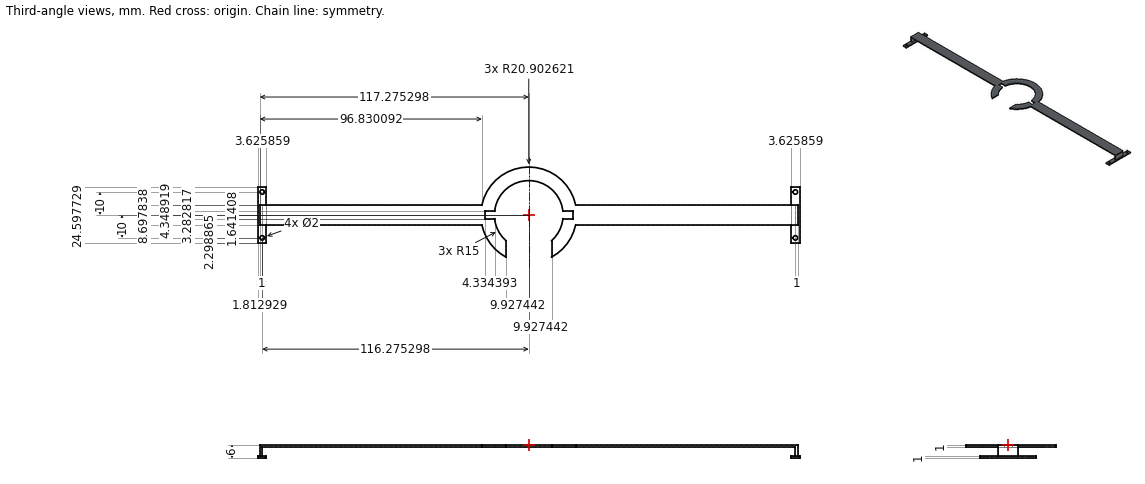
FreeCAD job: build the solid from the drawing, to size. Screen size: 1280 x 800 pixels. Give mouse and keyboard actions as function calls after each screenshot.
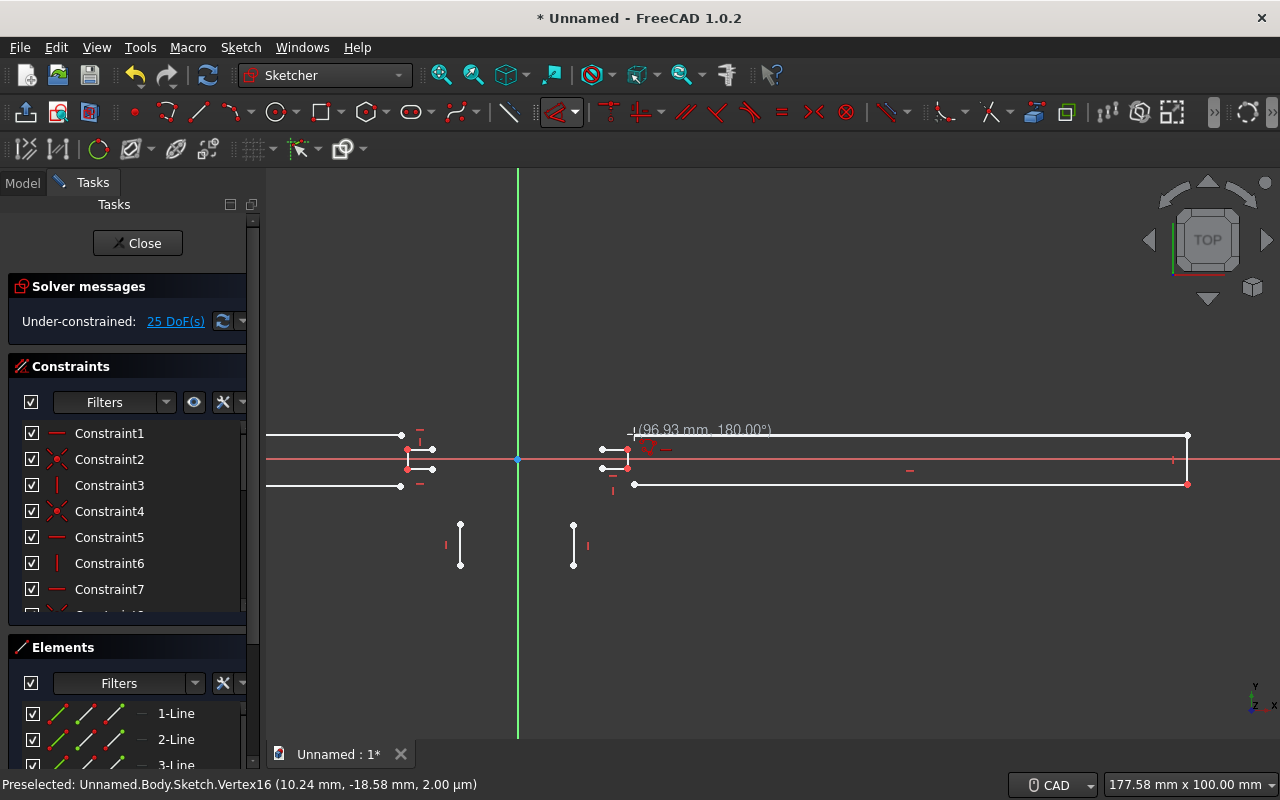
click(634, 434)
right_click(634, 434)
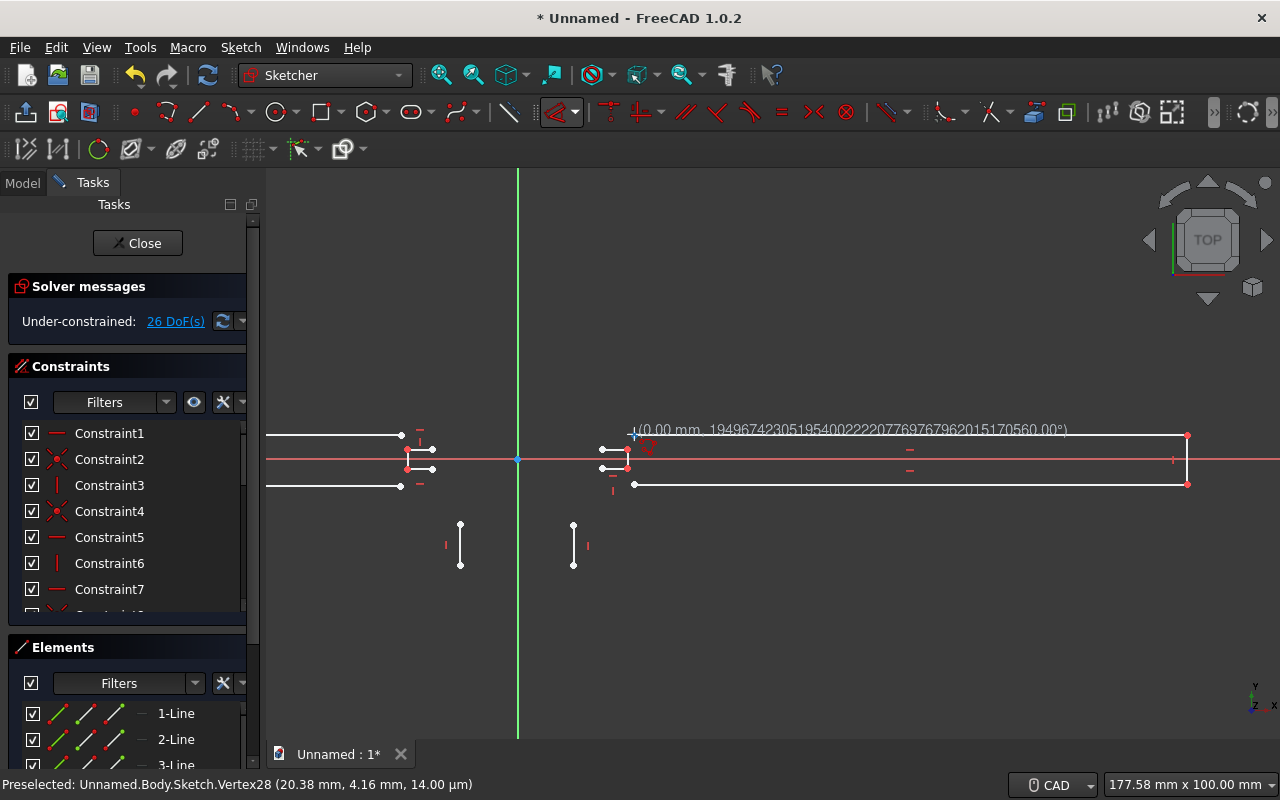
click(232, 112)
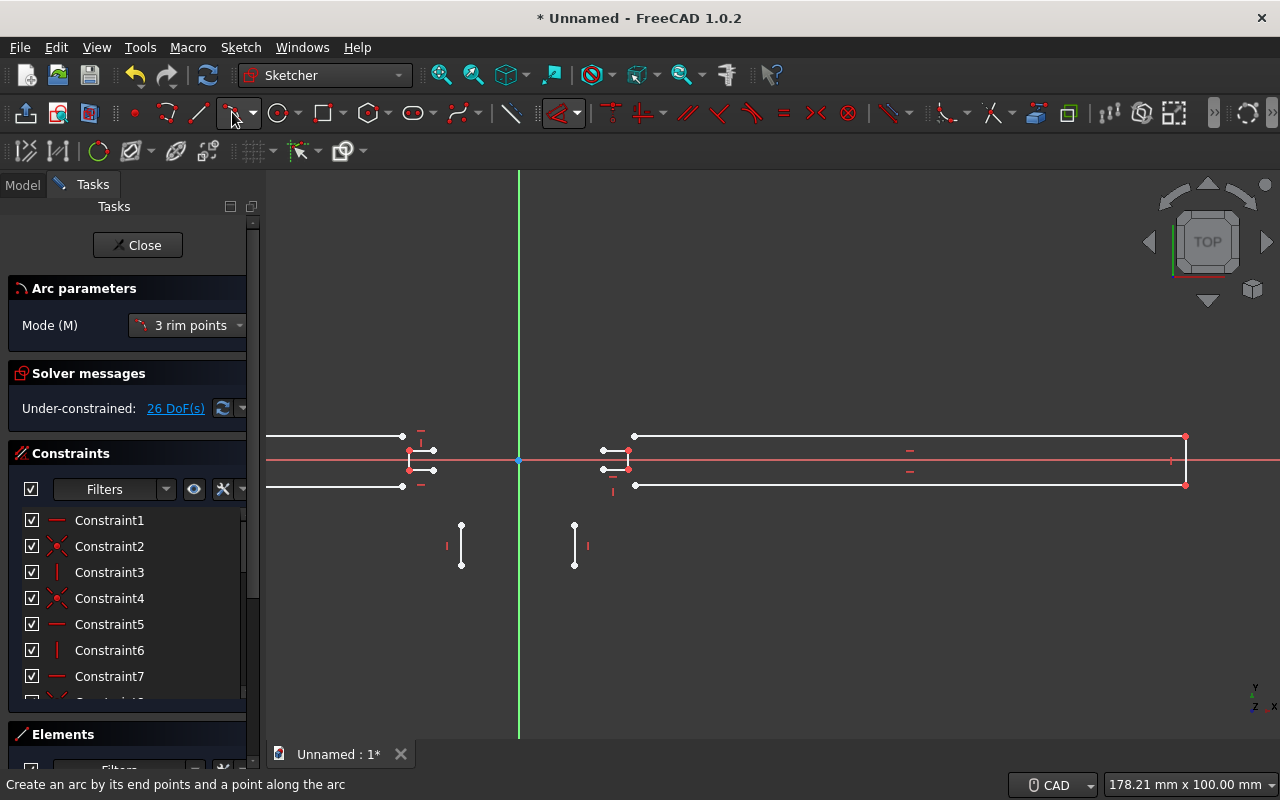
click(402, 487)
click(461, 566)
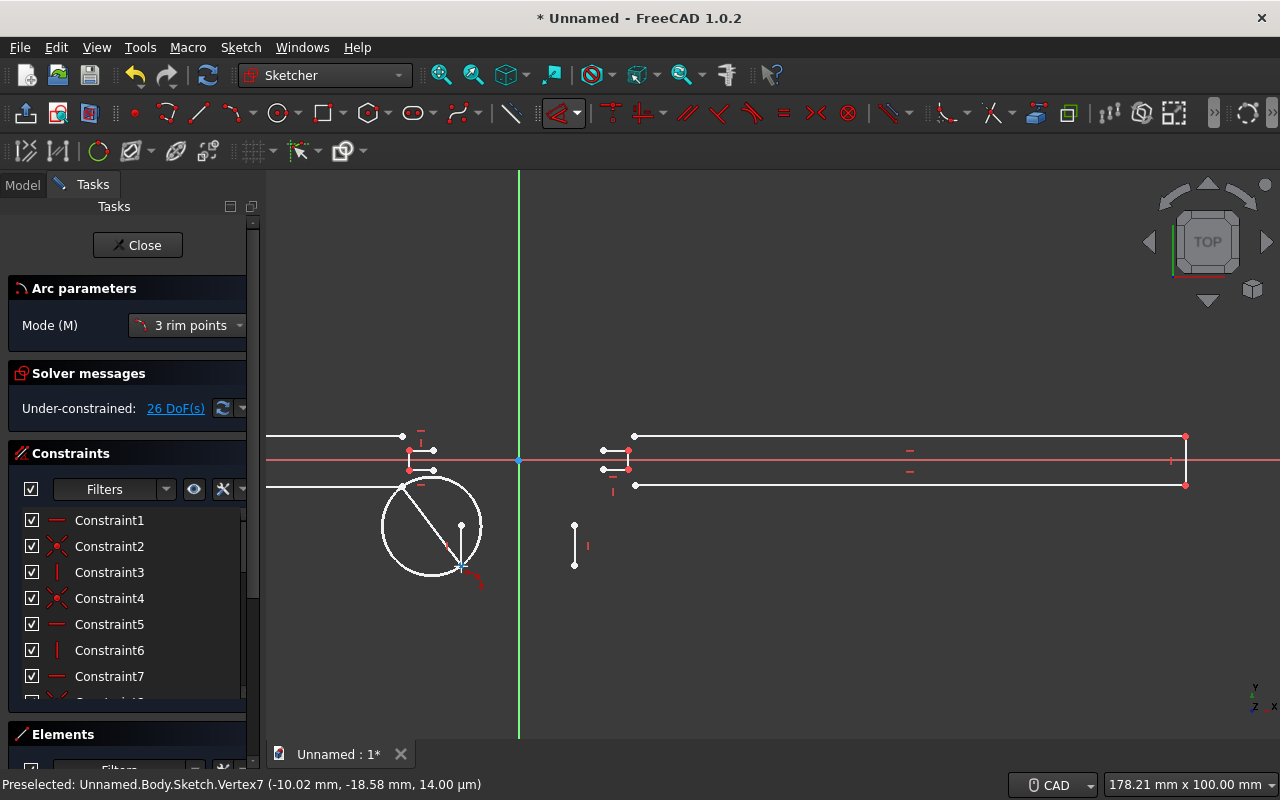
scroll(423, 531, up, 2)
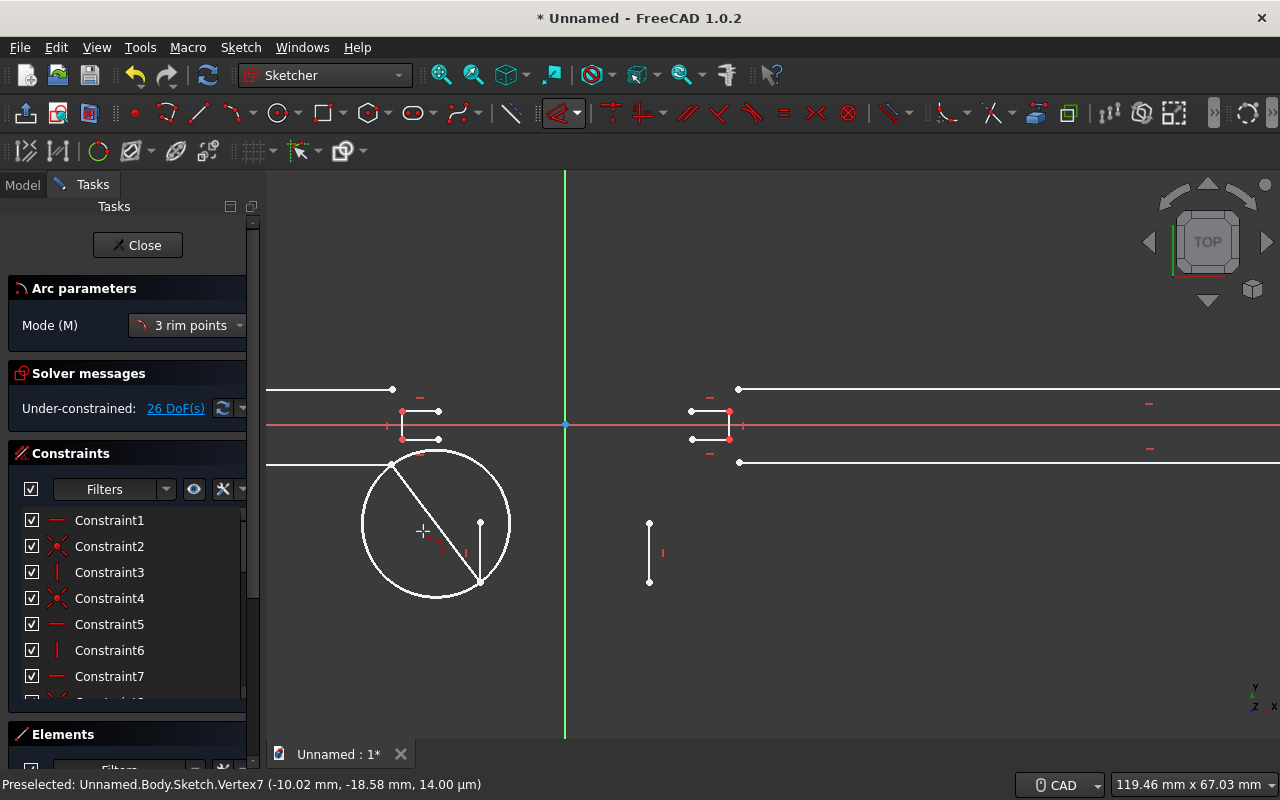
click(423, 531)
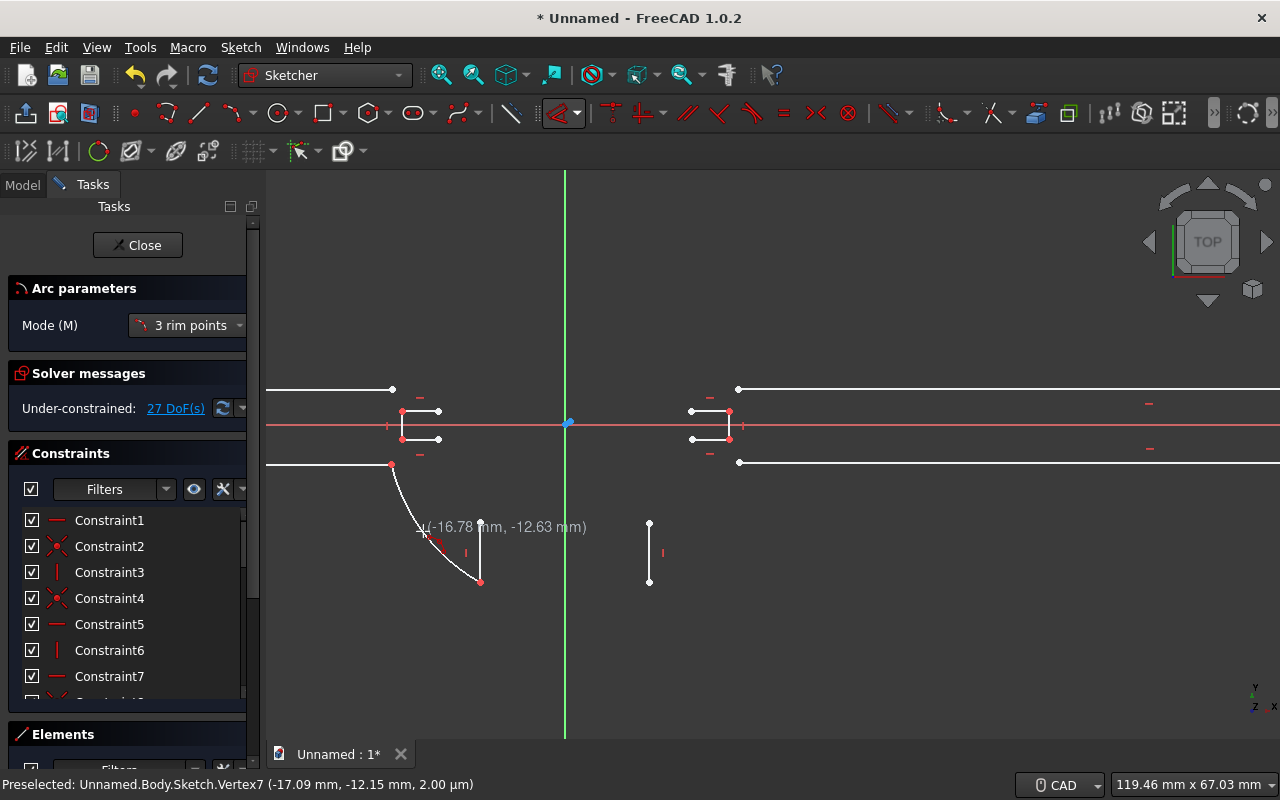
click(480, 523)
click(439, 440)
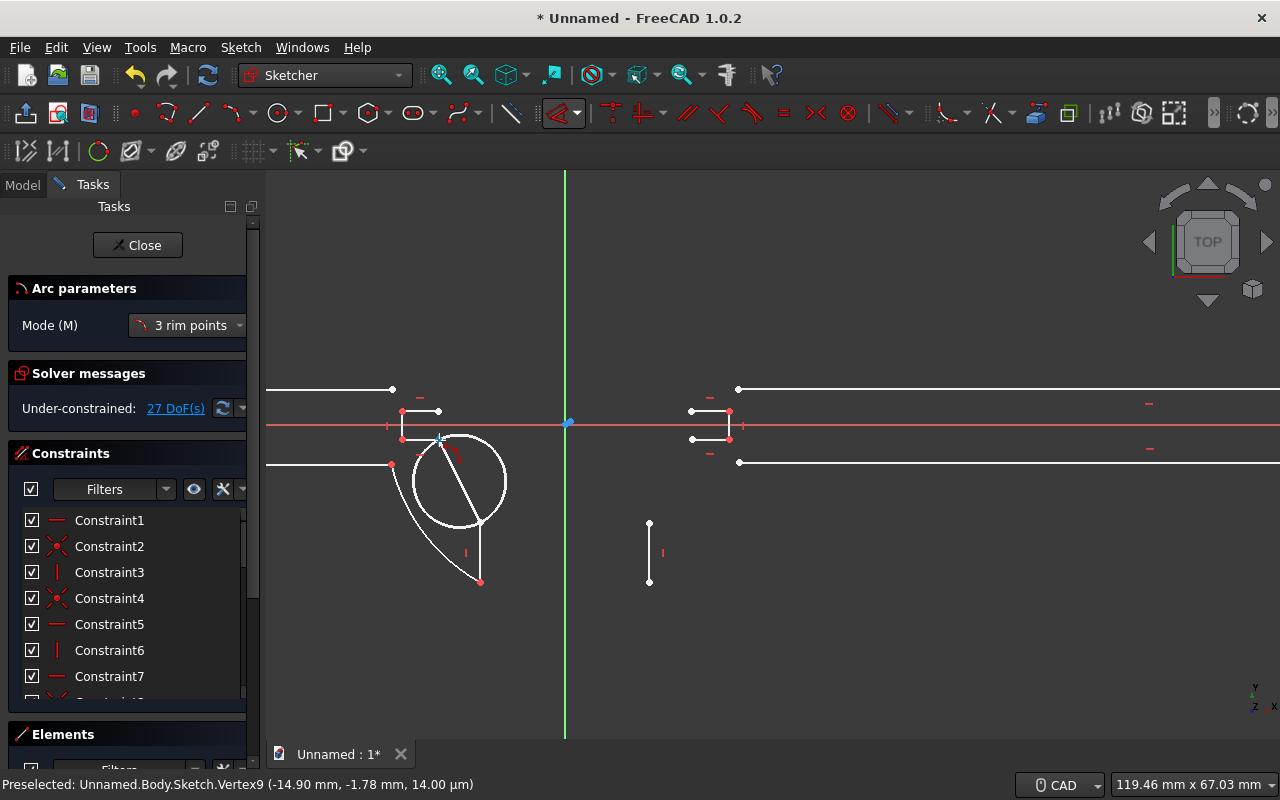
scroll(452, 483, up, 4)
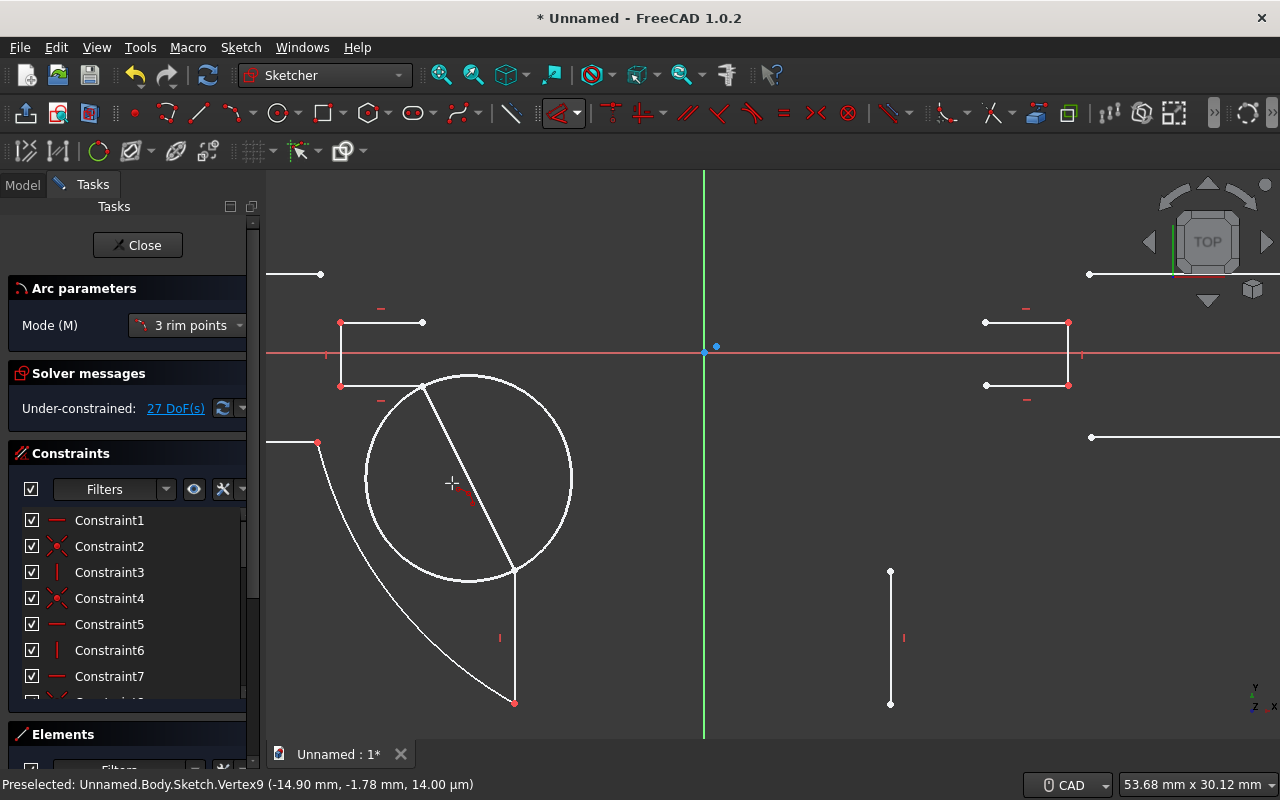
click(453, 483)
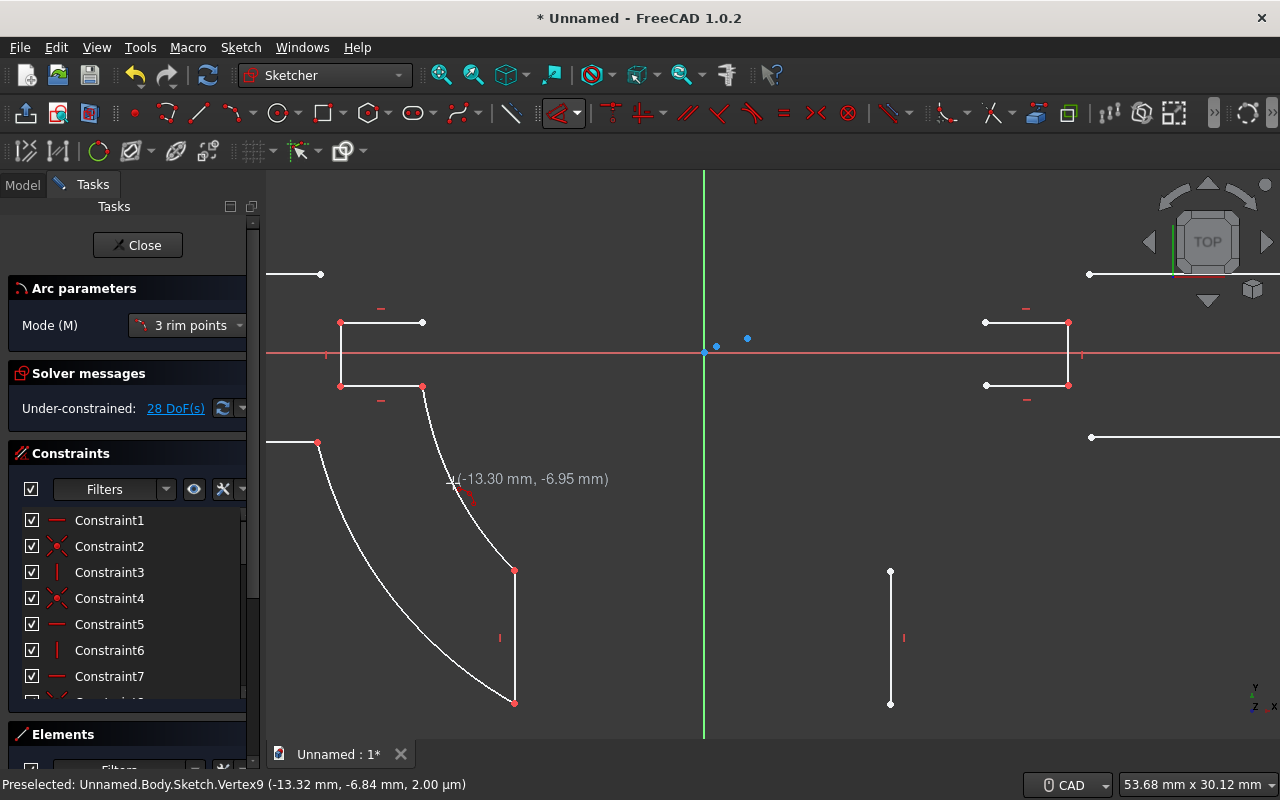
click(423, 323)
click(986, 323)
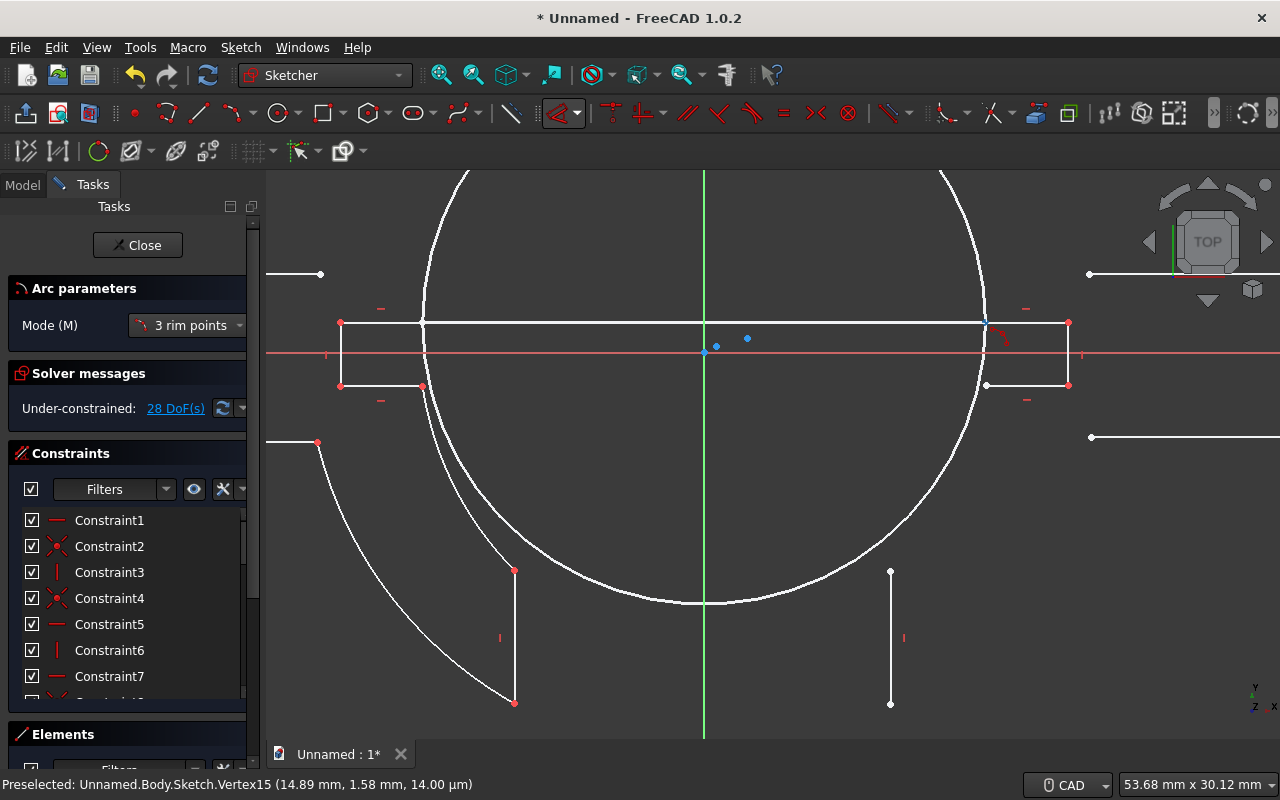
scroll(705, 474, down, 10)